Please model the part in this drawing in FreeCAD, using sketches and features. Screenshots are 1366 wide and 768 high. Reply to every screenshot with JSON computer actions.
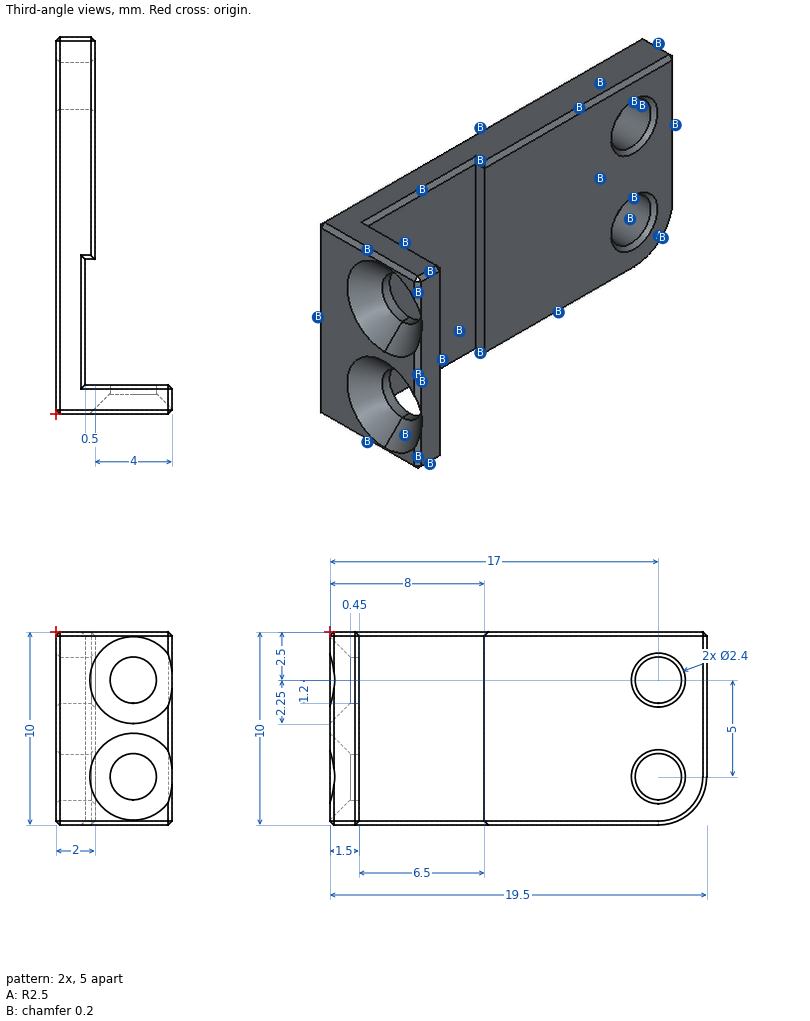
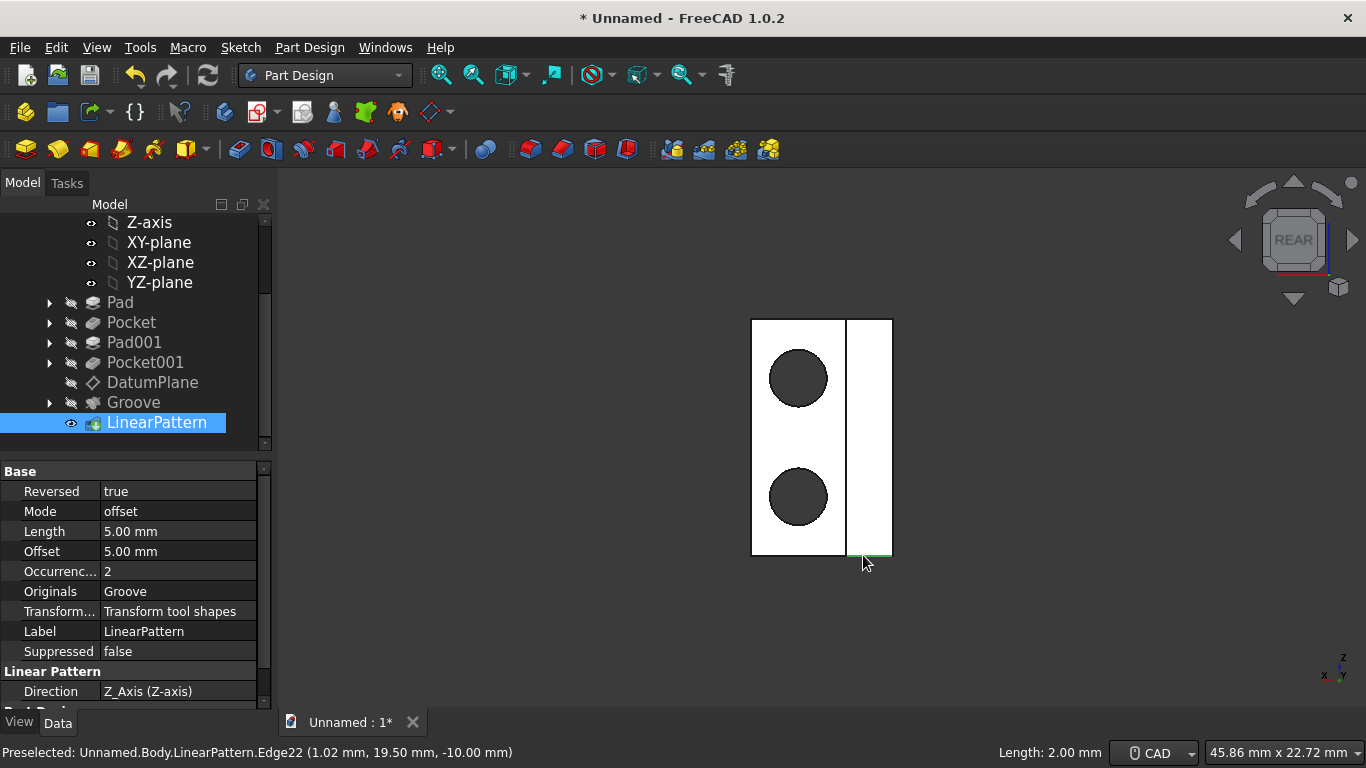
{"action": "left_click", "coordinate": [532, 150]}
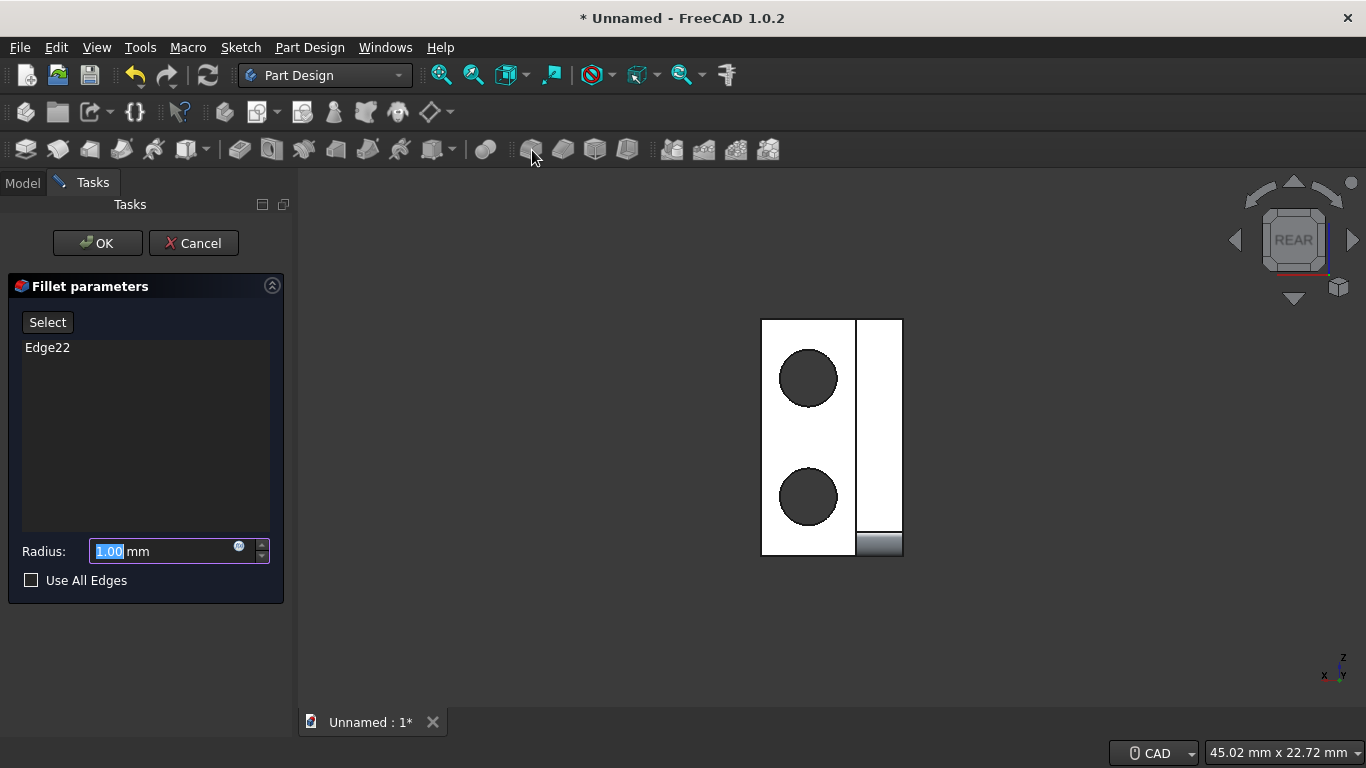
{"action": "type", "text": "2.5"}
{"action": "key", "text": "Tab"}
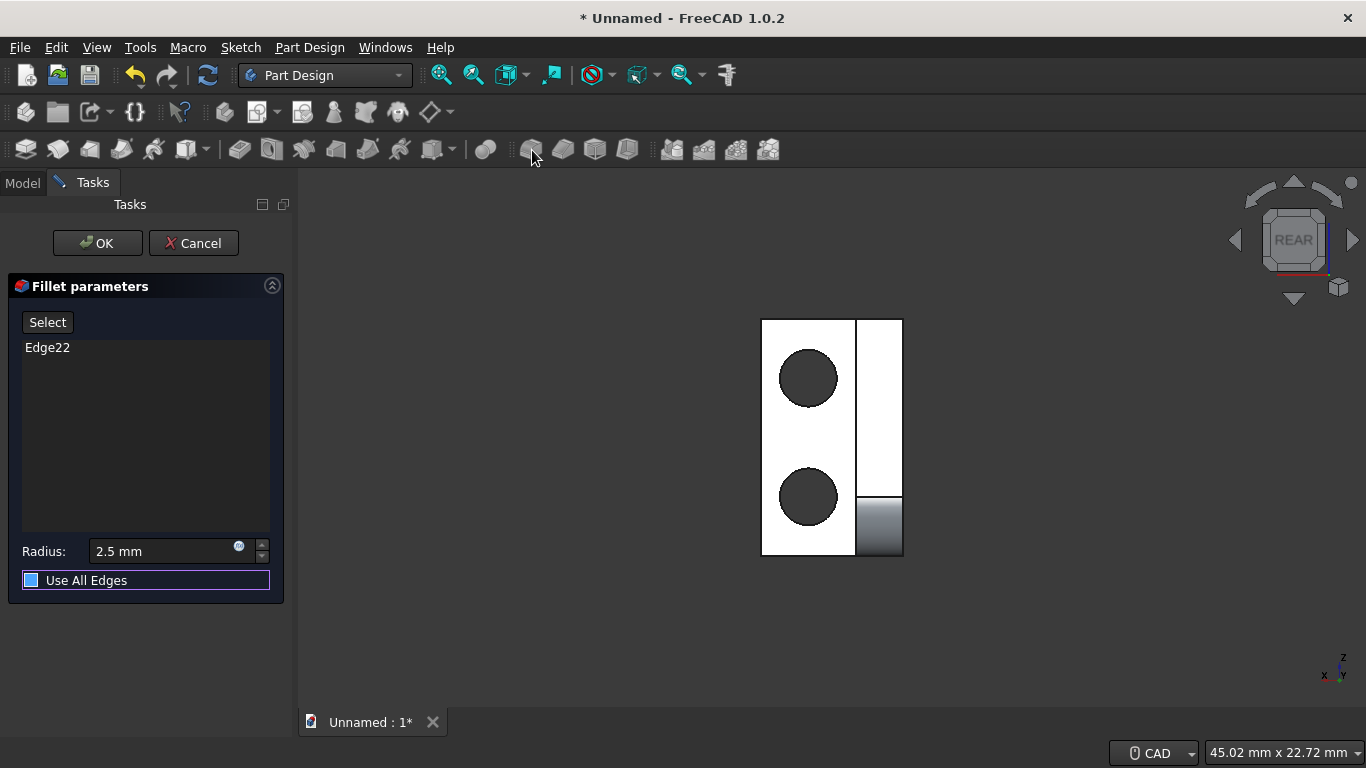
{"action": "left_click", "coordinate": [98, 243]}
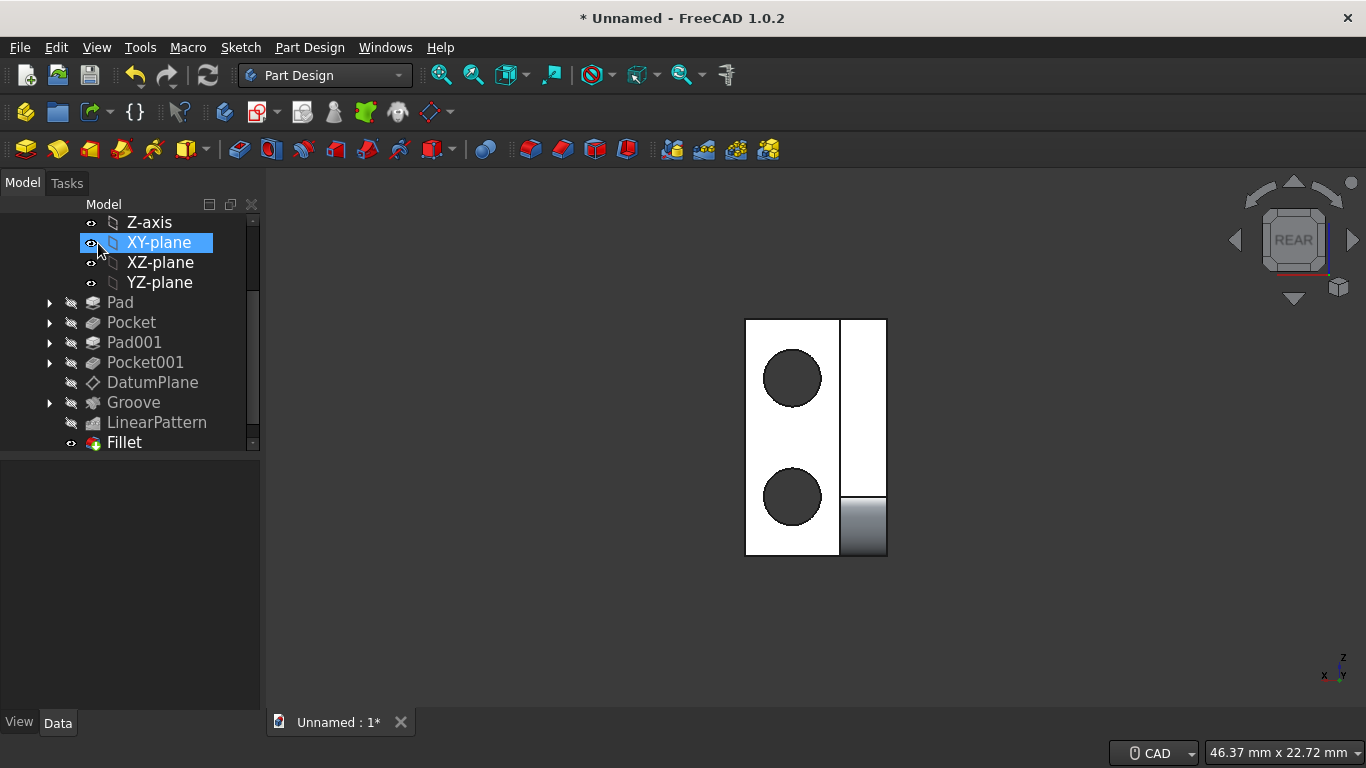
{"action": "left_click", "coordinate": [442, 76]}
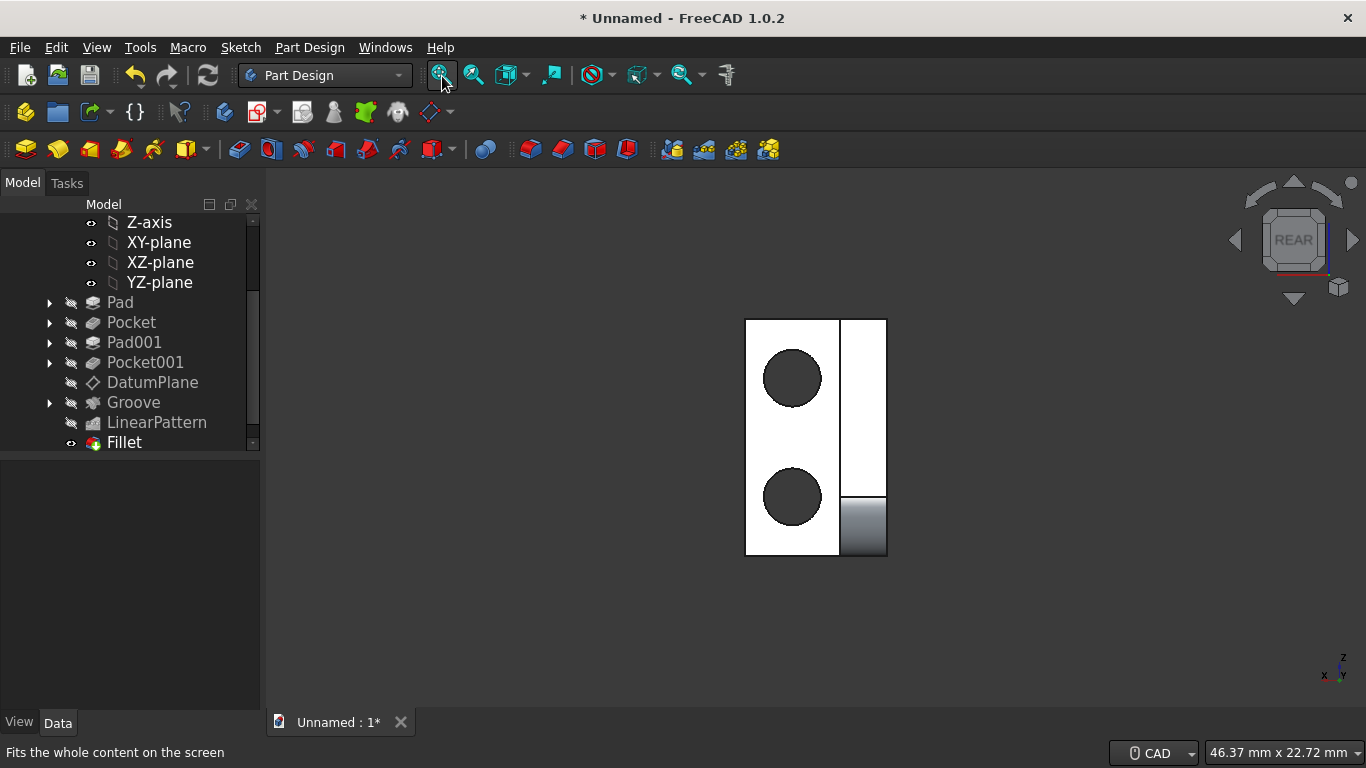
{"action": "left_click", "coordinate": [840, 407]}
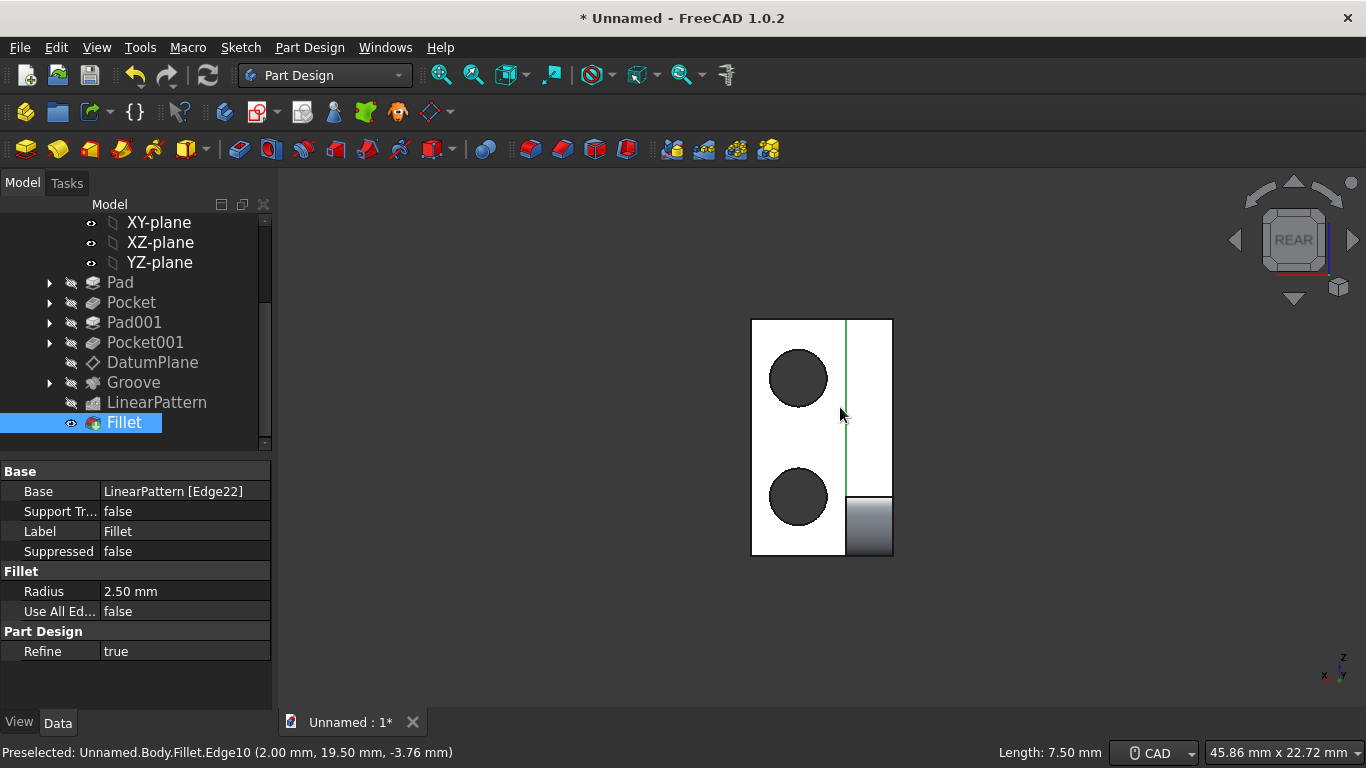
{"action": "left_click", "coordinate": [846, 538], "text": "ctrl"}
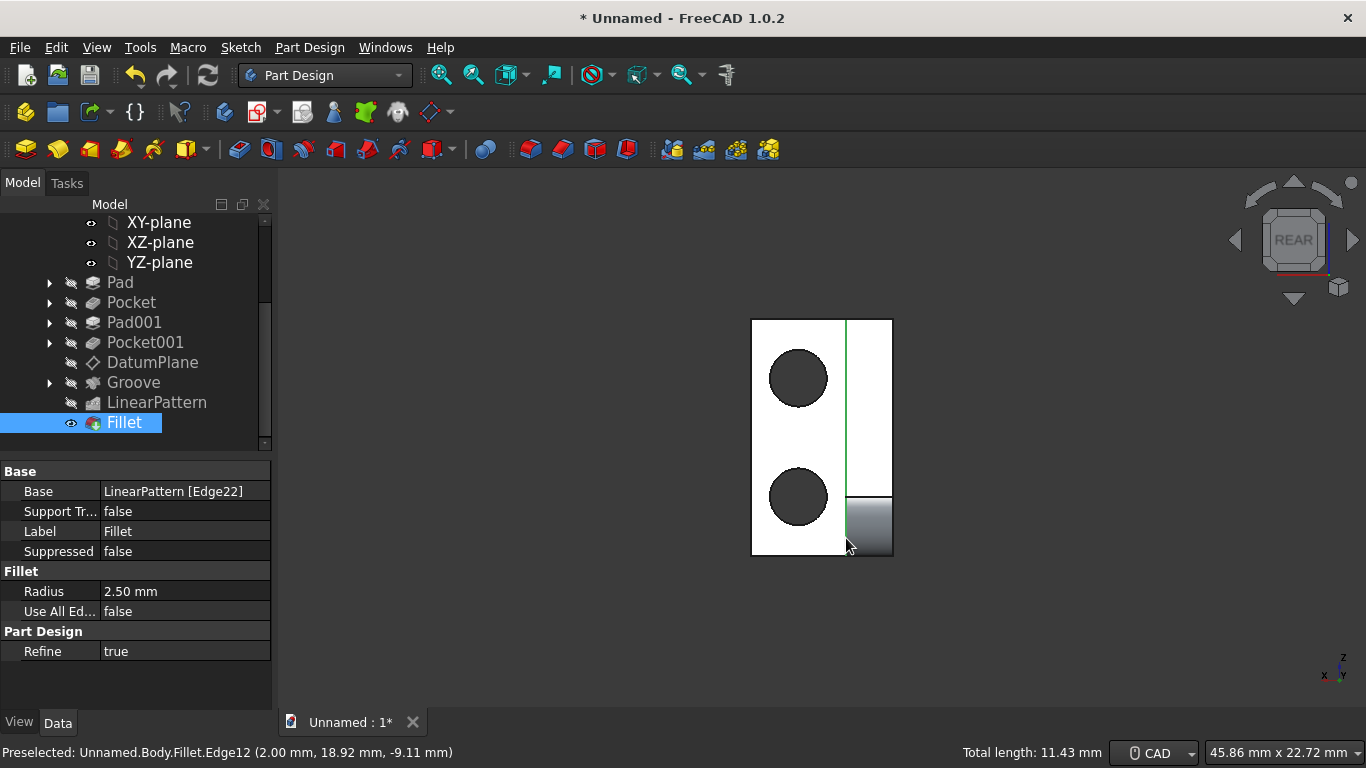
{"action": "left_click", "coordinate": [804, 555], "text": "ctrl"}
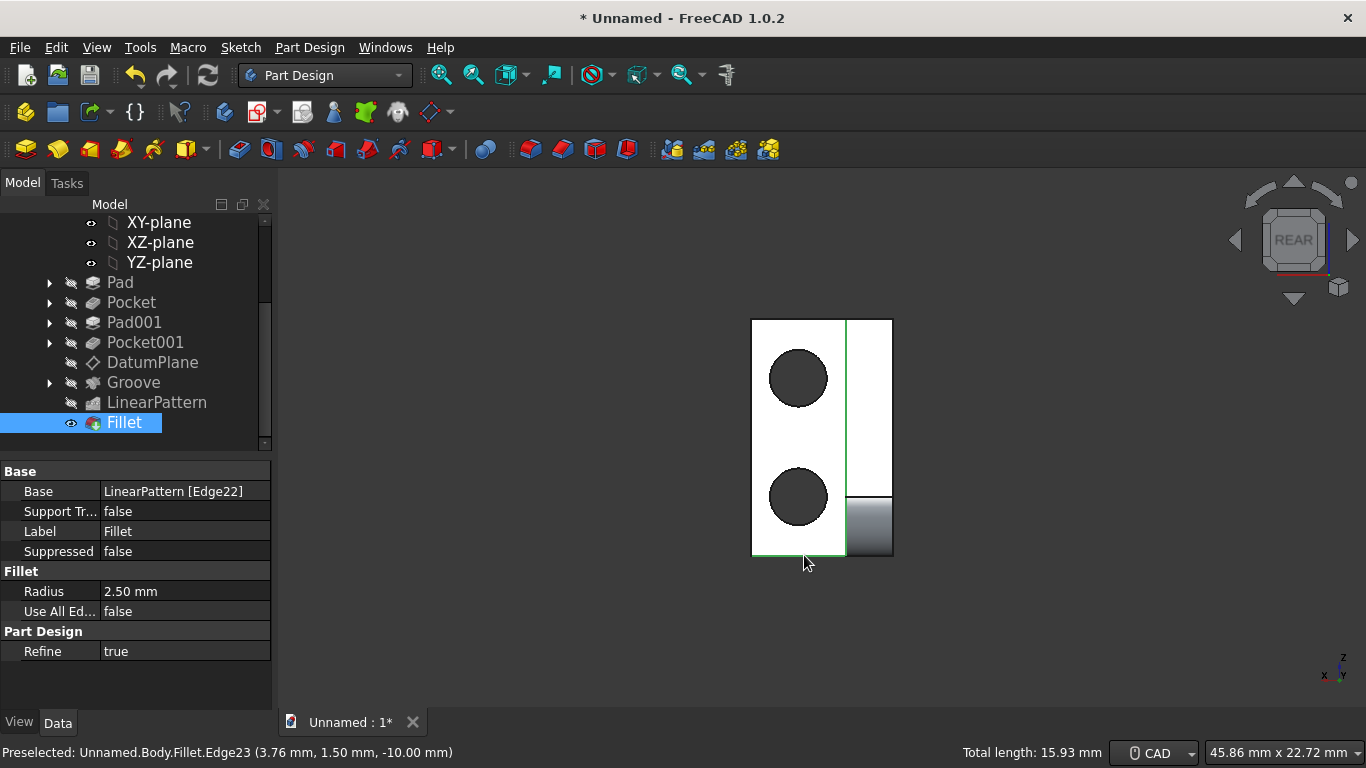
{"action": "left_click", "coordinate": [751, 437], "text": "ctrl"}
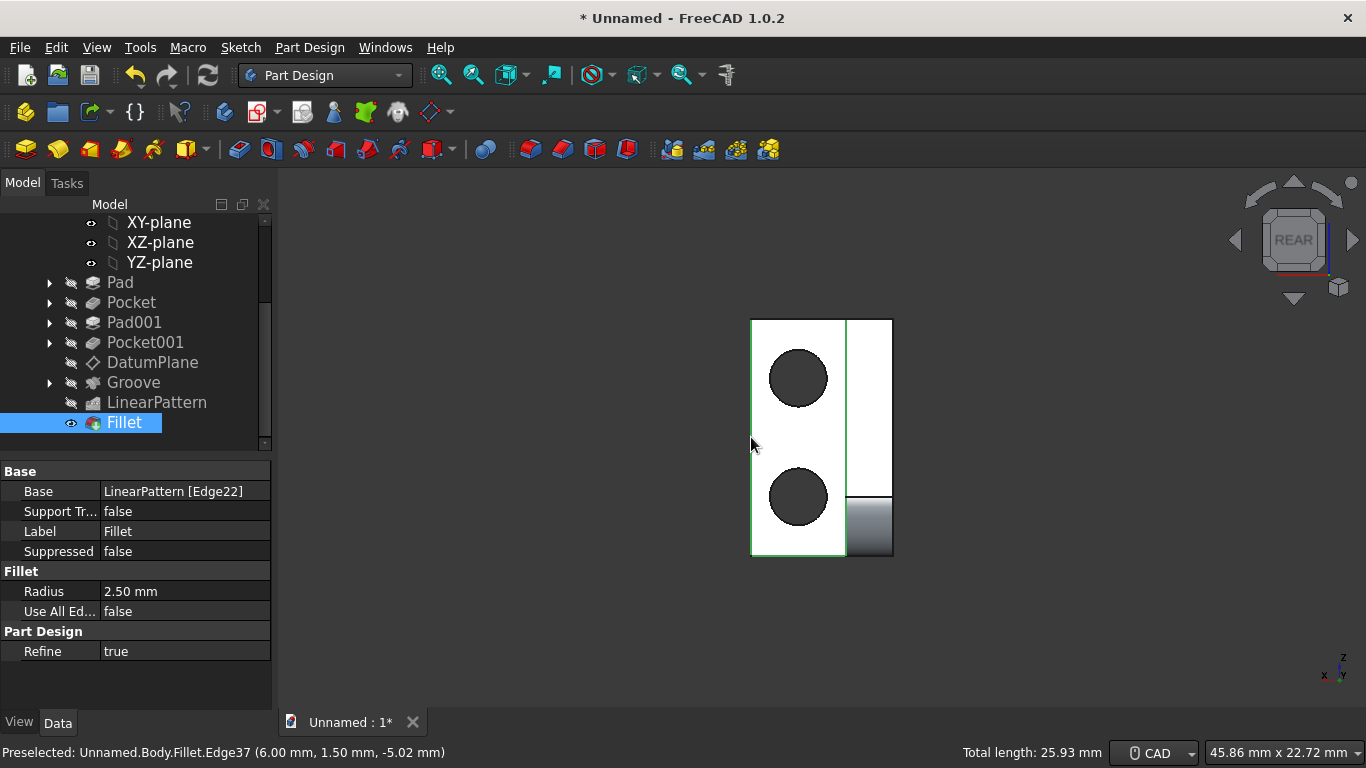
{"action": "key", "text": "0"}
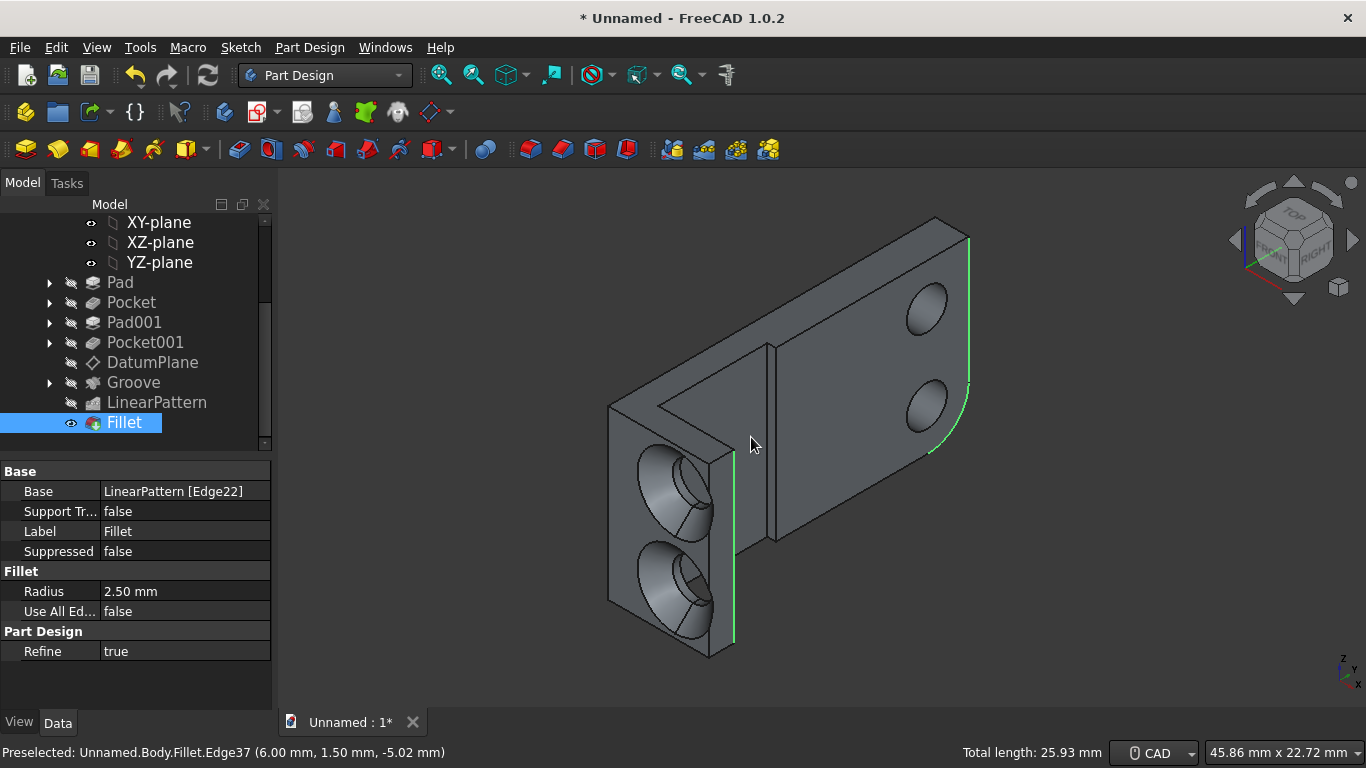
{"action": "left_click", "coordinate": [933, 242], "text": "ctrl"}